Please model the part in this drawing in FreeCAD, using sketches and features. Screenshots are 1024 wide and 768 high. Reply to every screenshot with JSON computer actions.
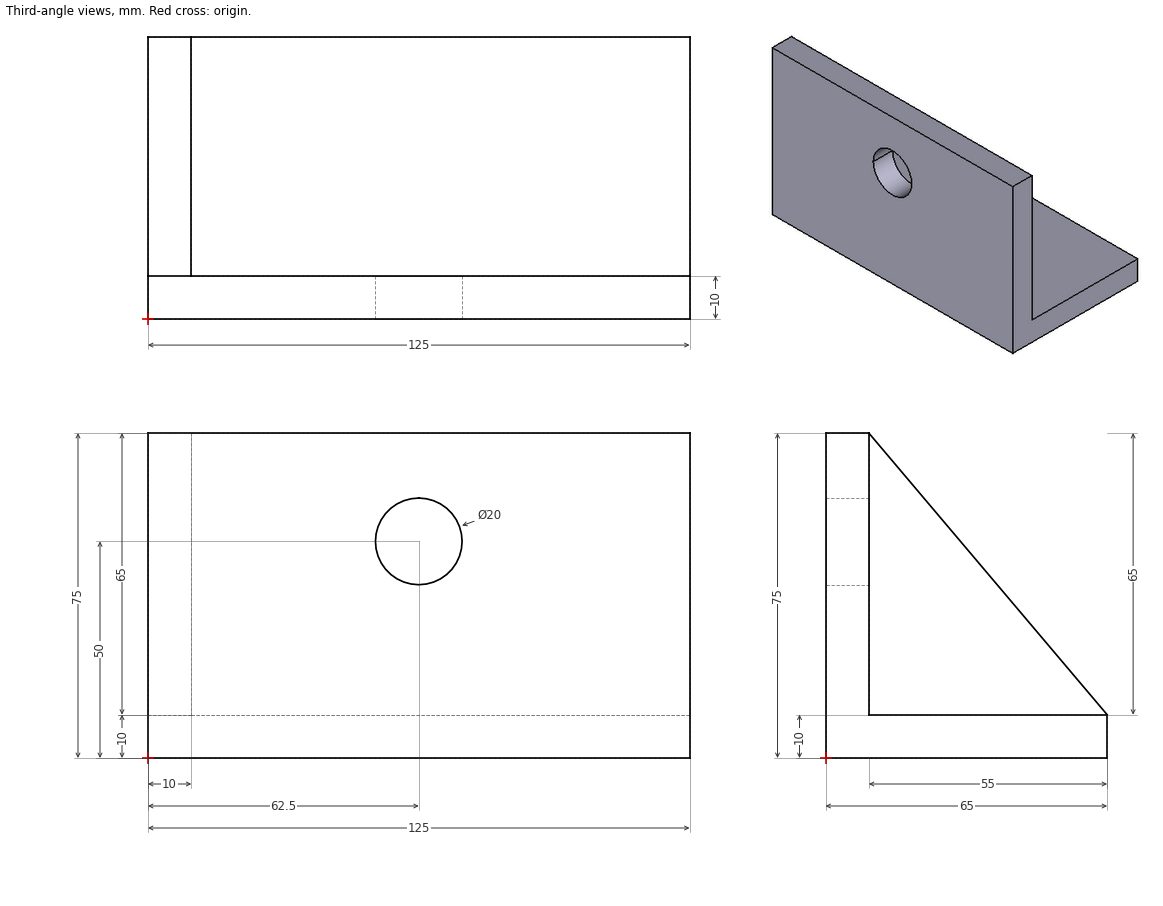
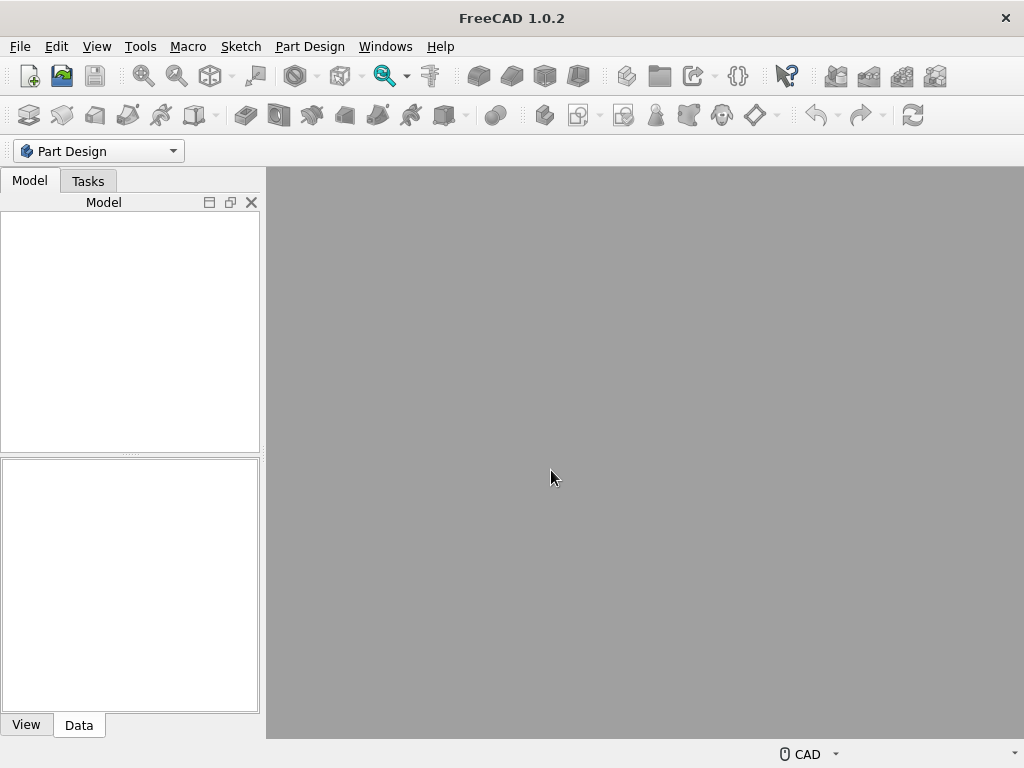
{"action": "left_click", "coordinate": [29, 76]}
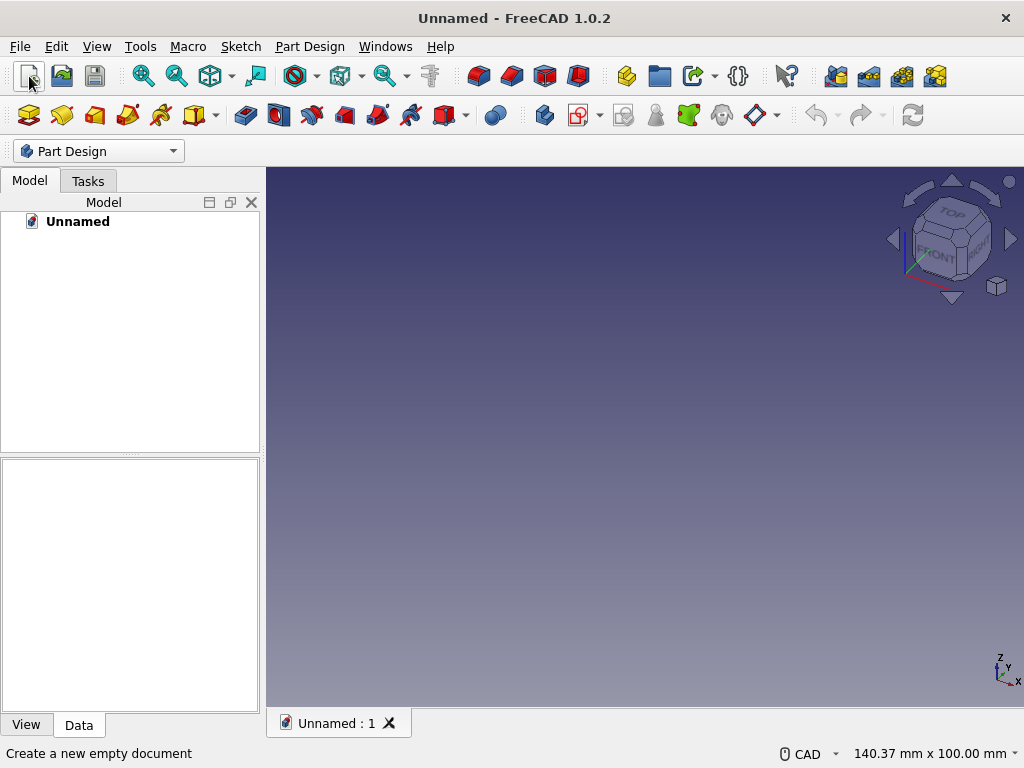
{"action": "left_click", "coordinate": [578, 116]}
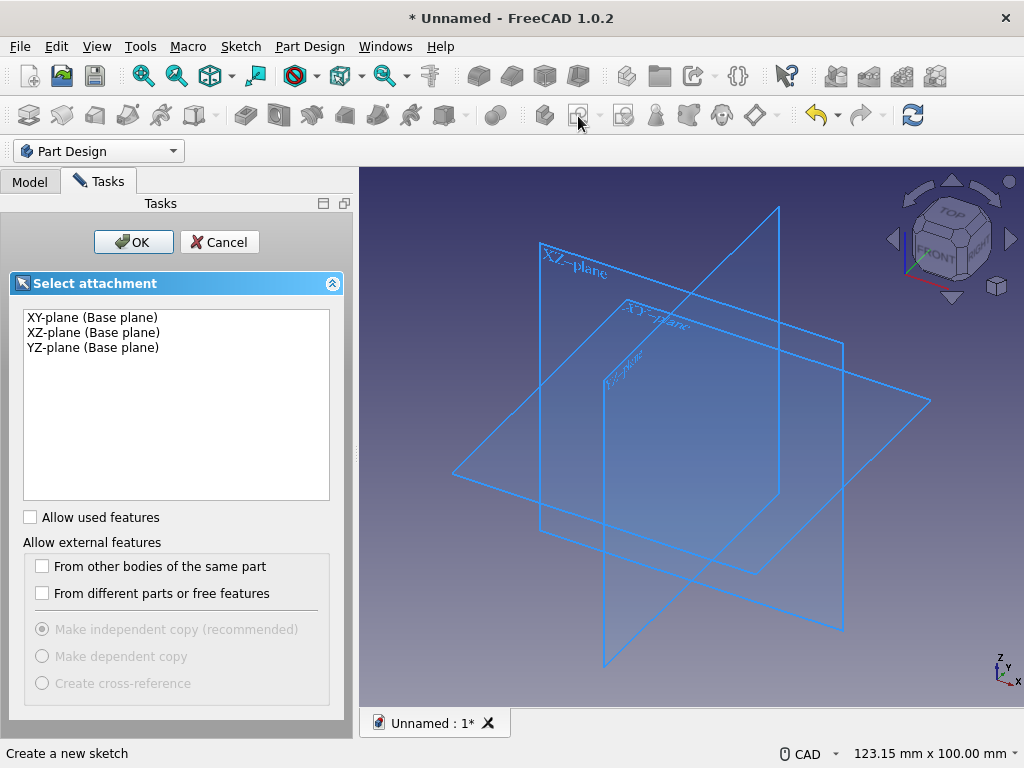
{"action": "left_click", "coordinate": [84, 318]}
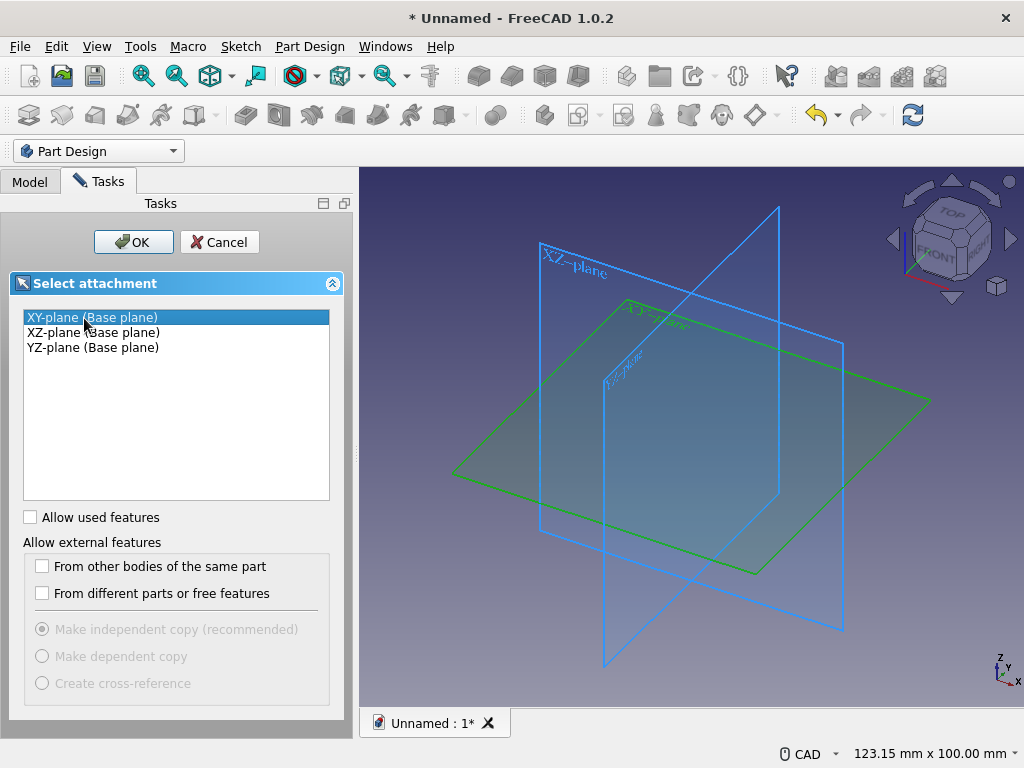
{"action": "left_click", "coordinate": [134, 242]}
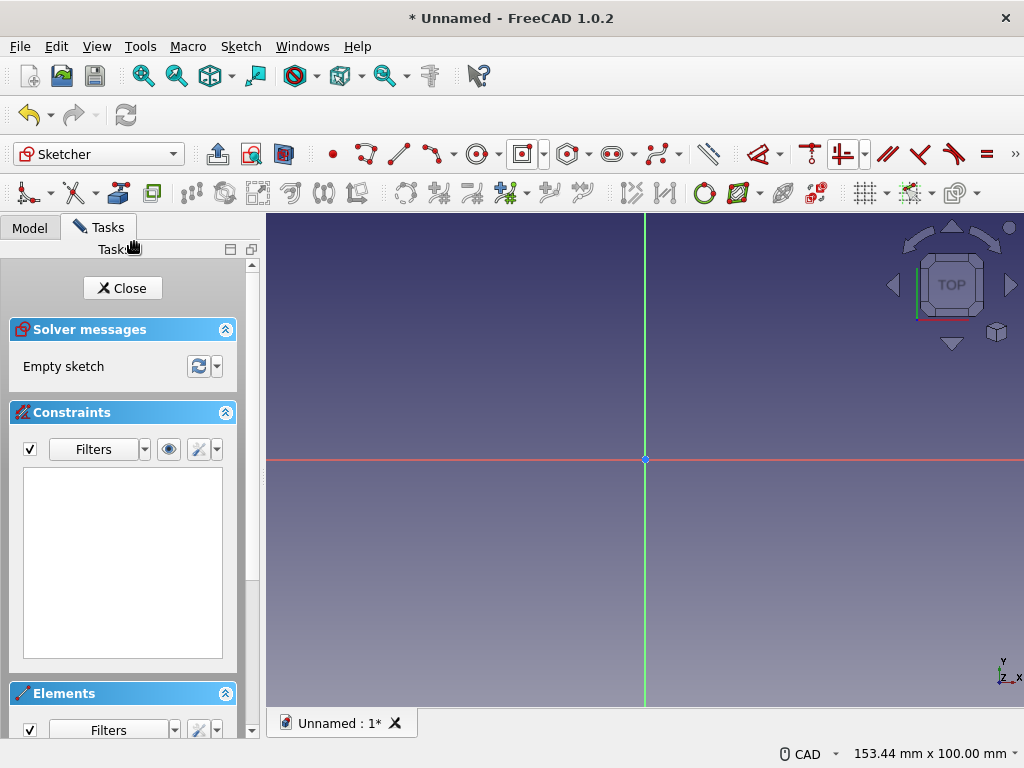
{"action": "scroll", "coordinate": [294, 490], "scroll_direction": "down", "scroll_amount": 3}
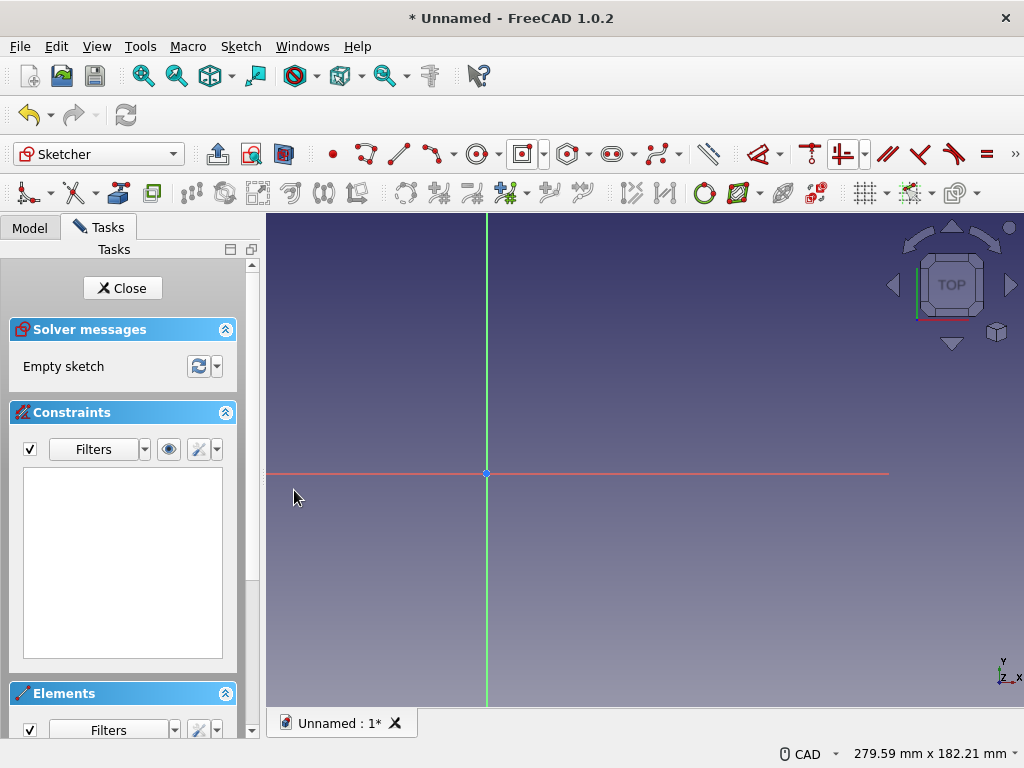
{"action": "left_click", "coordinate": [544, 154]}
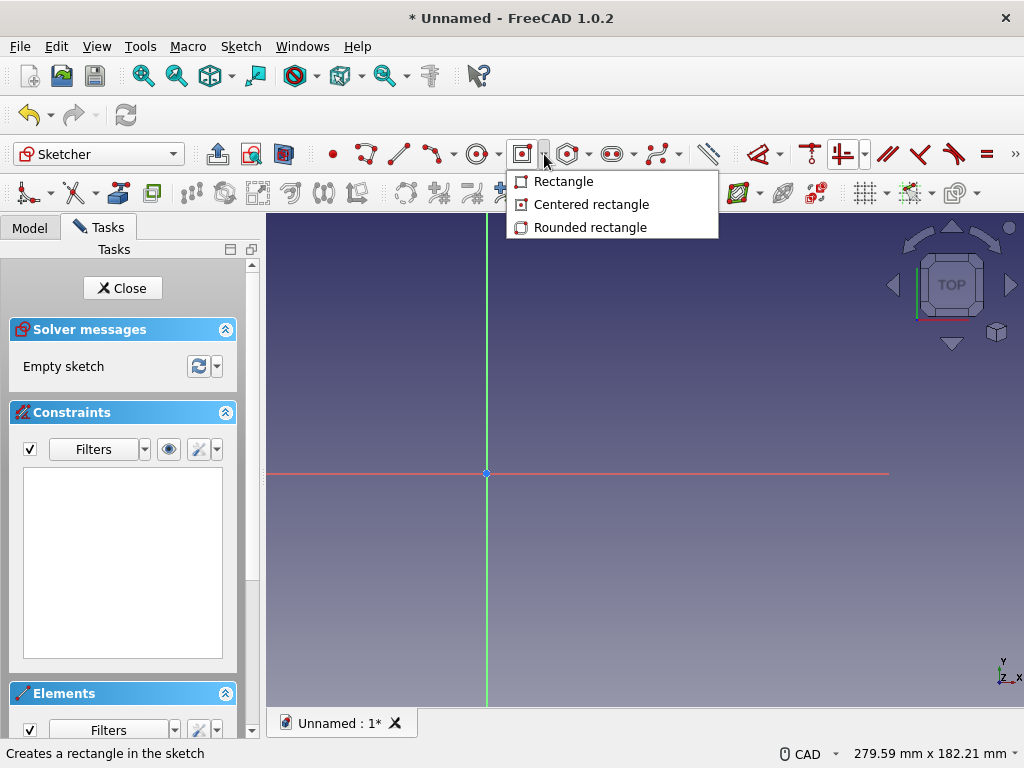
{"action": "left_click", "coordinate": [612, 182]}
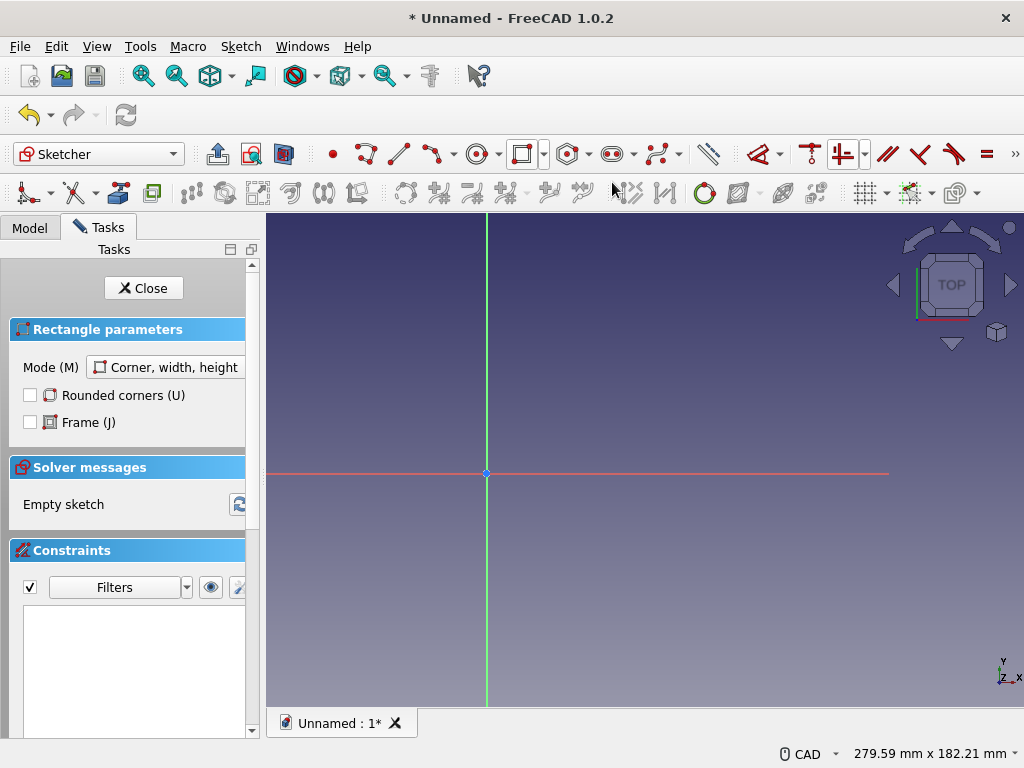
{"action": "left_click", "coordinate": [487, 474]}
{"action": "left_click", "coordinate": [826, 447]}
{"action": "key", "text": "Escape"}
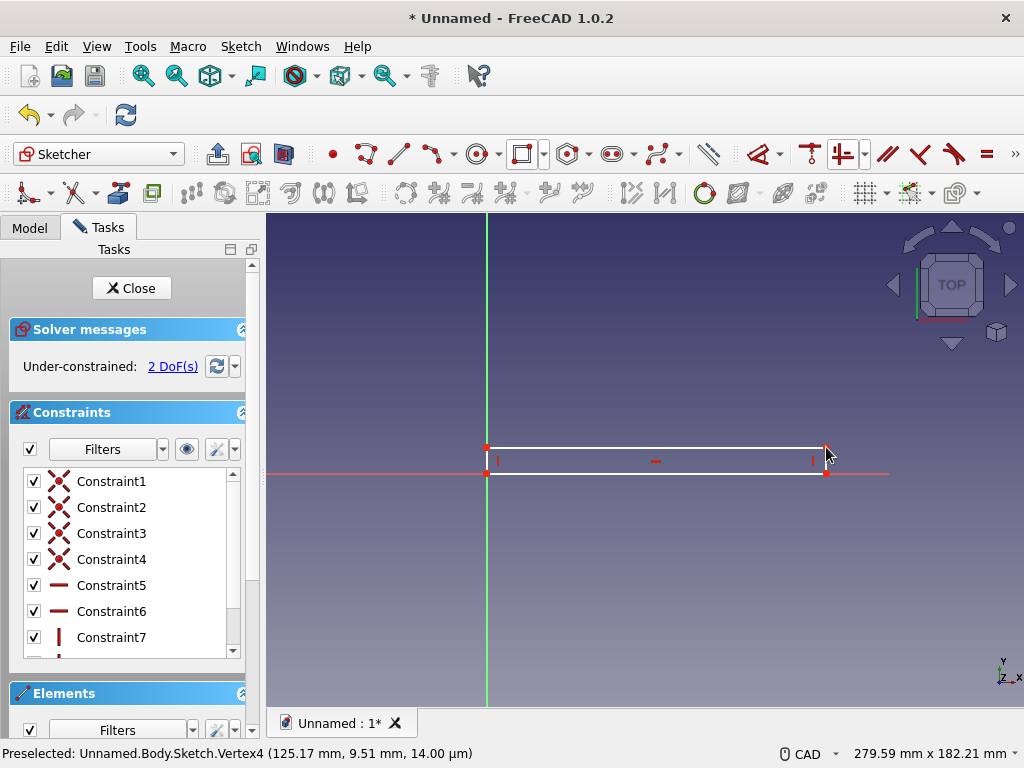
{"action": "scroll", "coordinate": [826, 463], "scroll_direction": "up", "scroll_amount": 2}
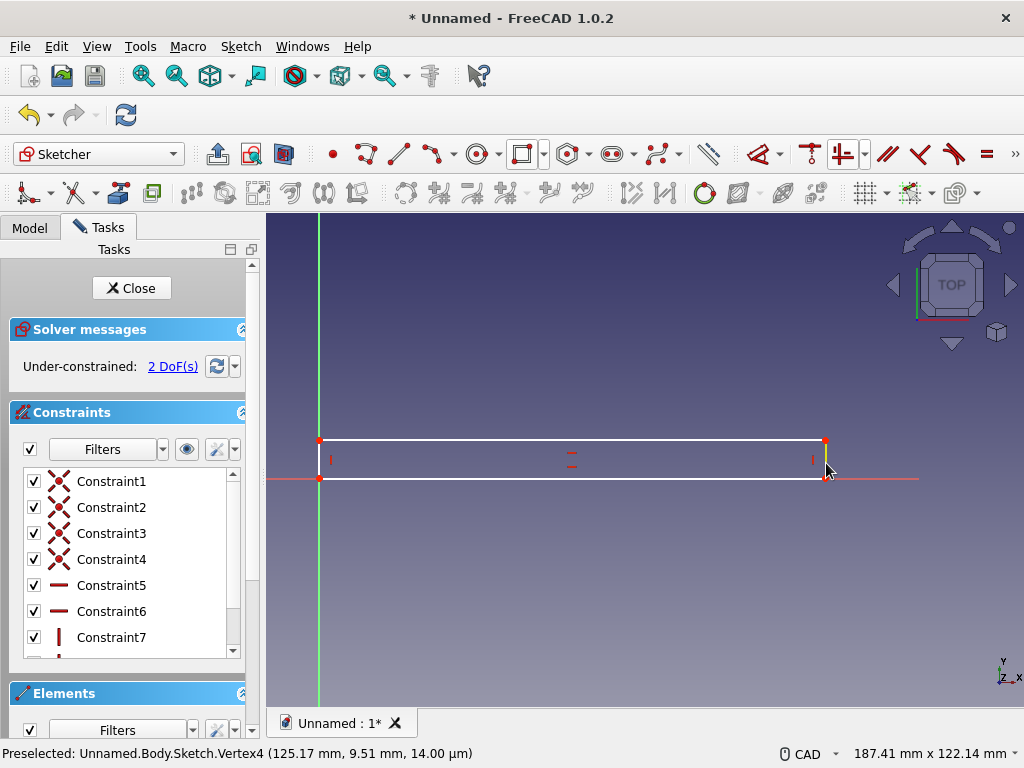
{"action": "left_click", "coordinate": [826, 463]}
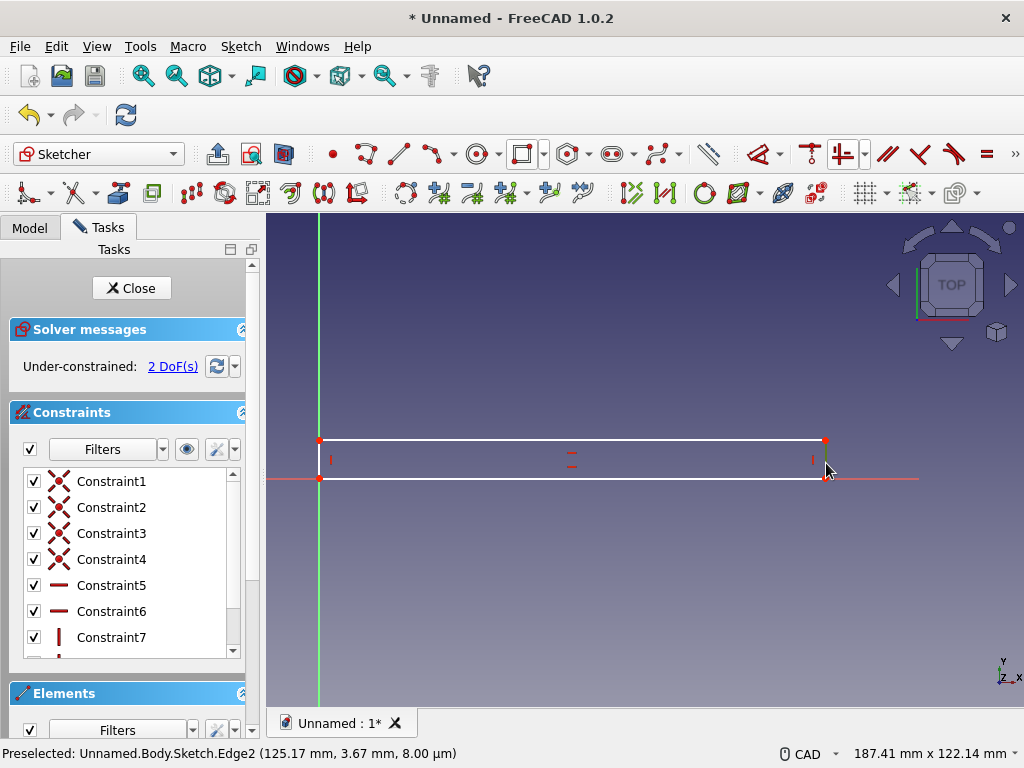
{"action": "left_click", "coordinate": [780, 154]}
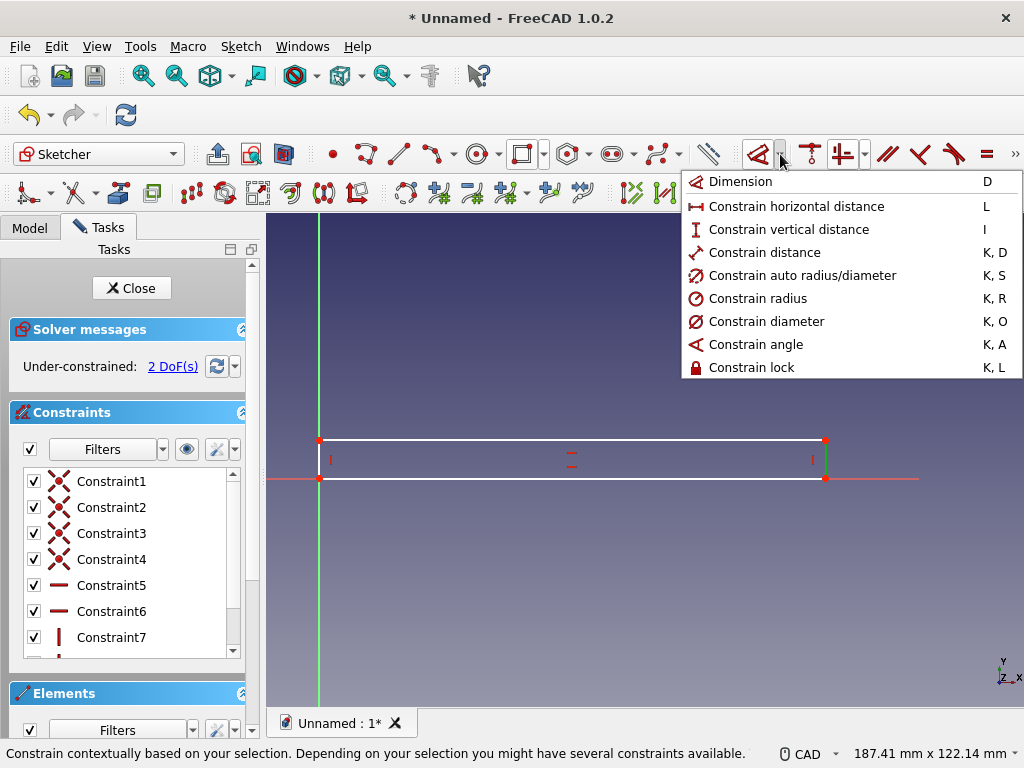
{"action": "left_click", "coordinate": [852, 230]}